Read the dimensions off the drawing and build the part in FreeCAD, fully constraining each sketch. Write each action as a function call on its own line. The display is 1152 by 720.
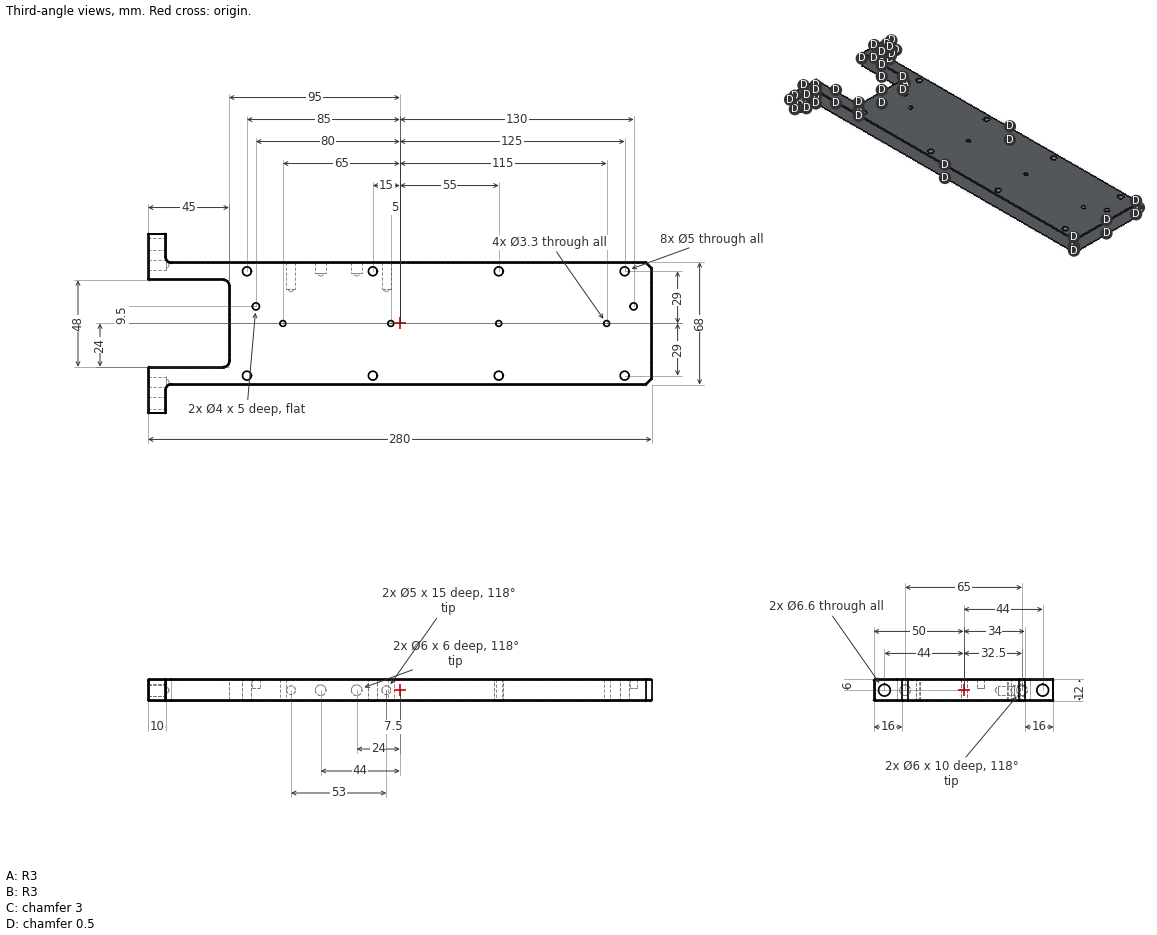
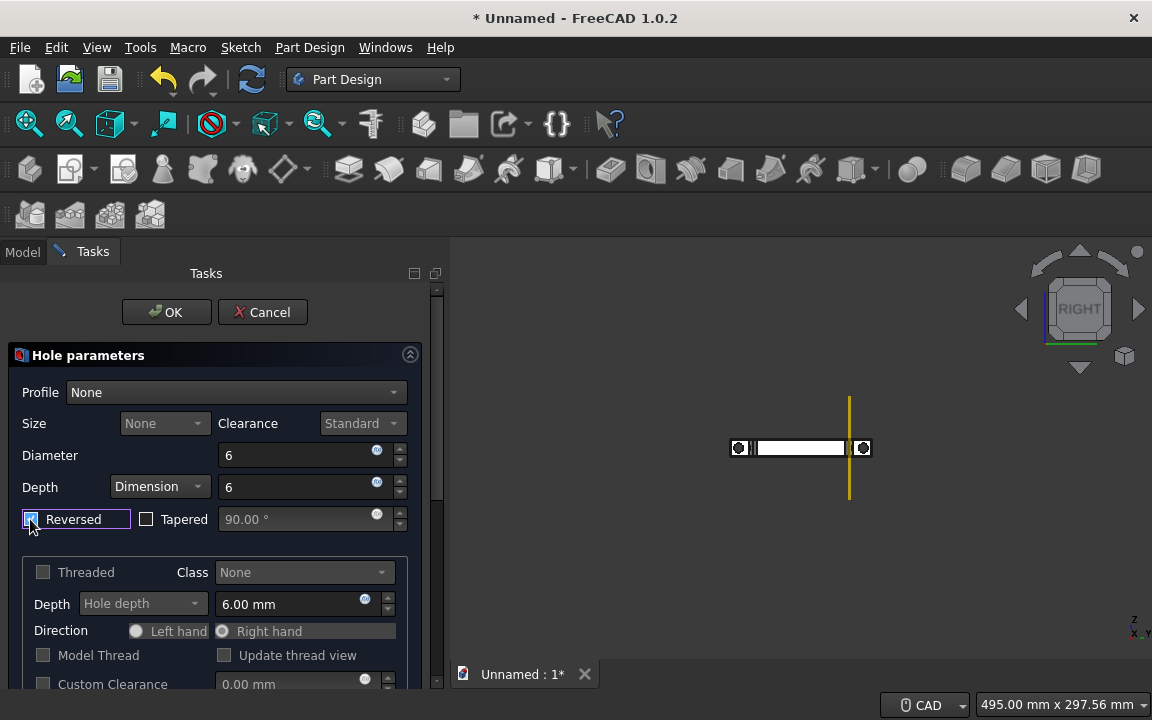
click(167, 312)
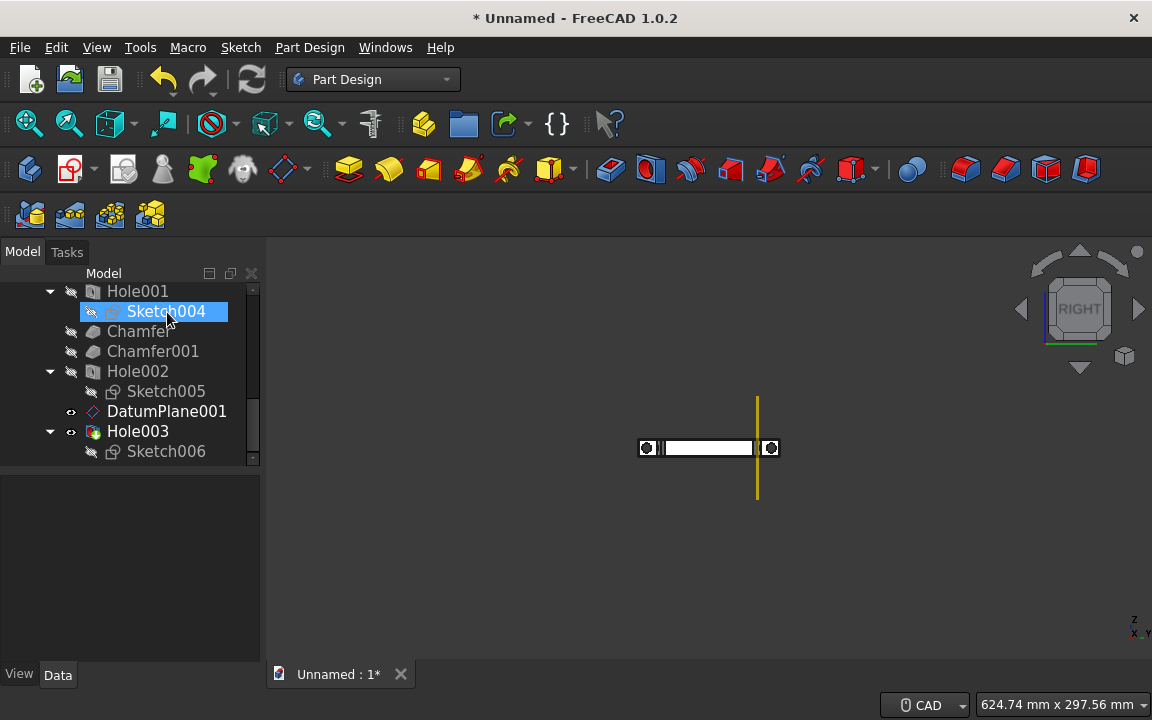
click(116, 412)
key(space)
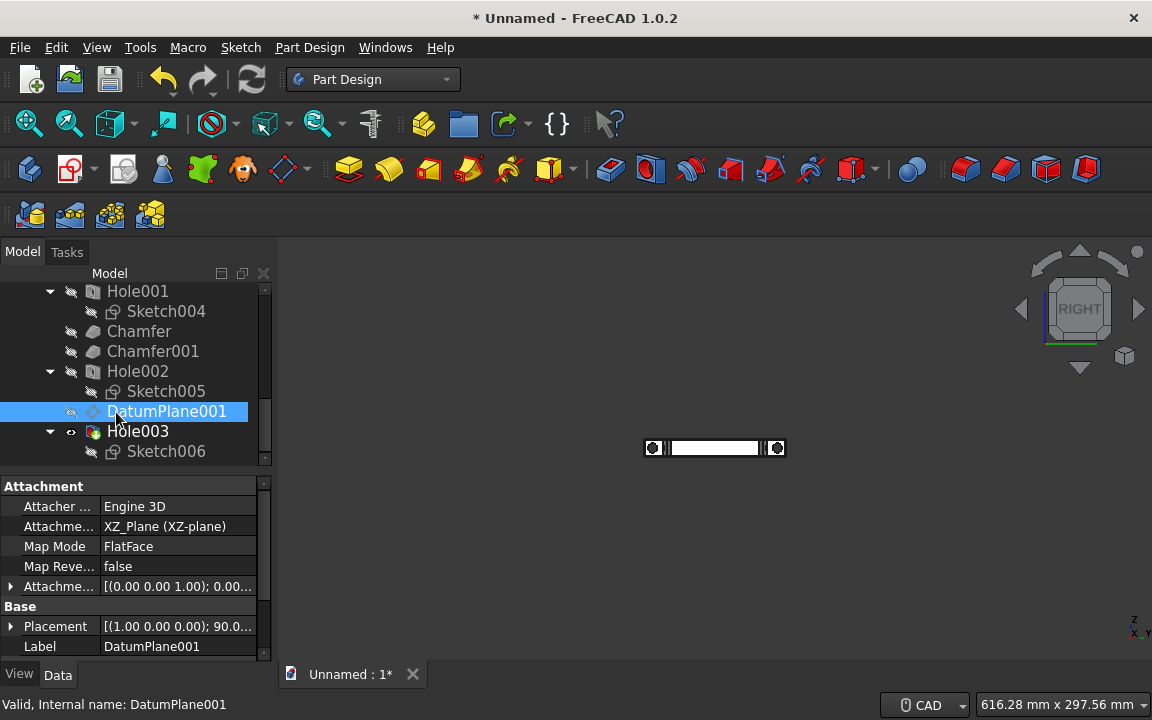
click(30, 124)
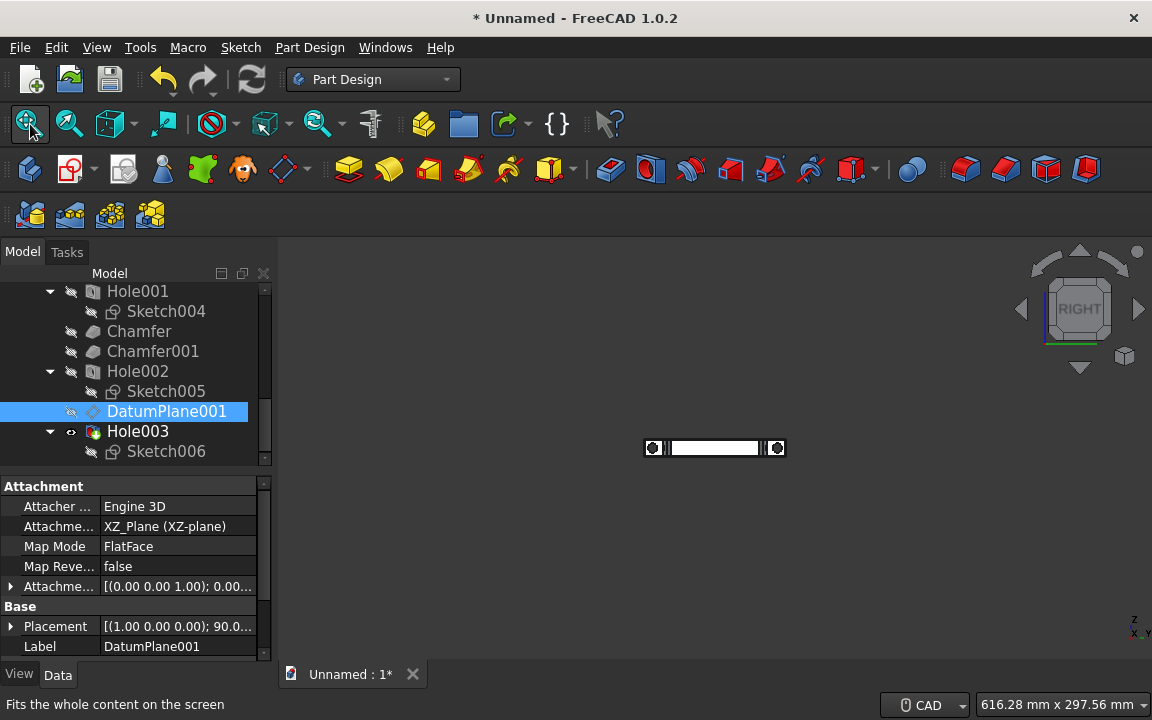
key(4)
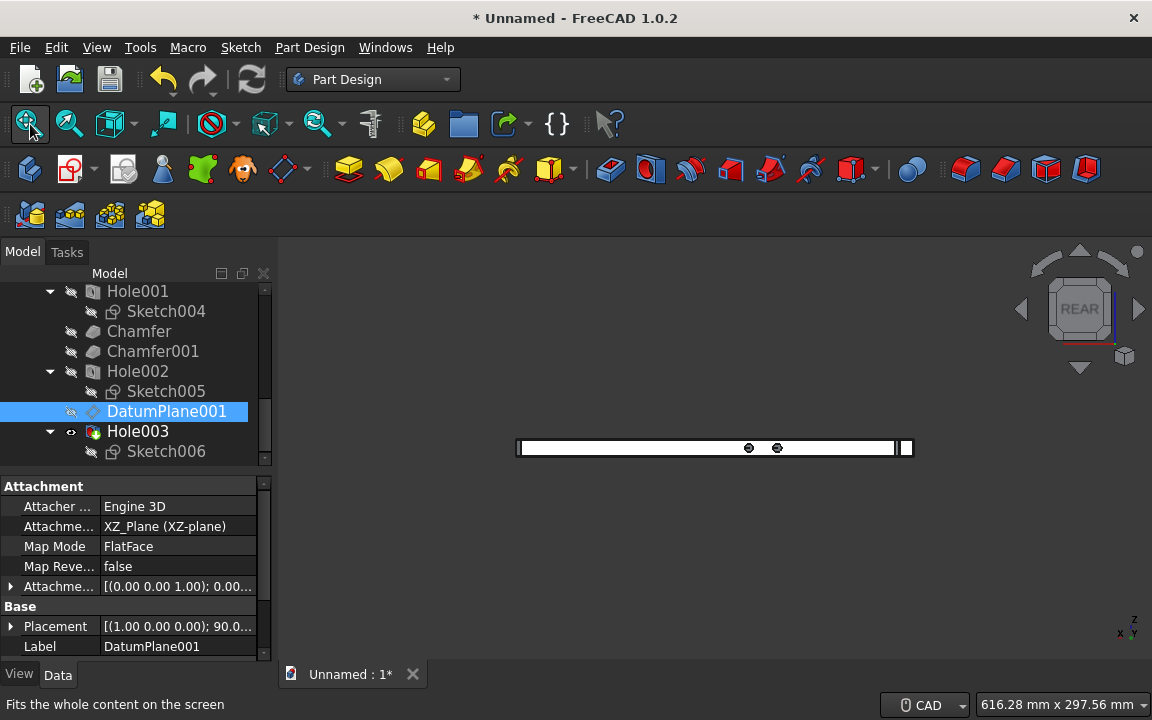
key(2)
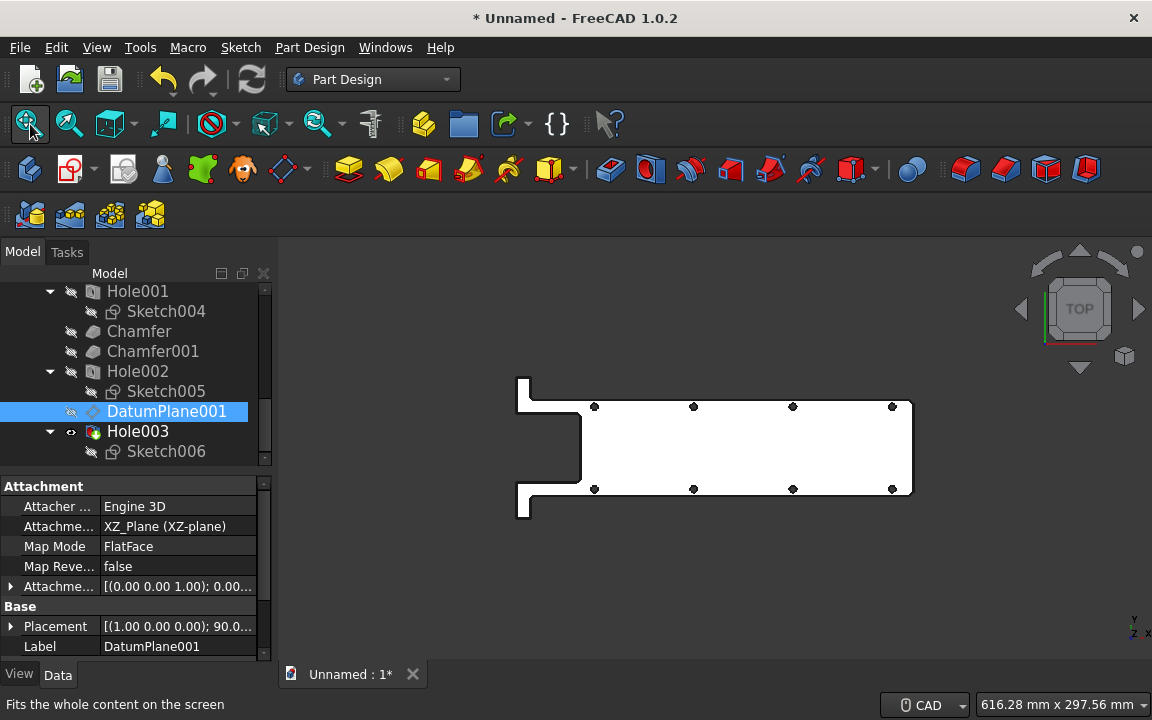
key(3)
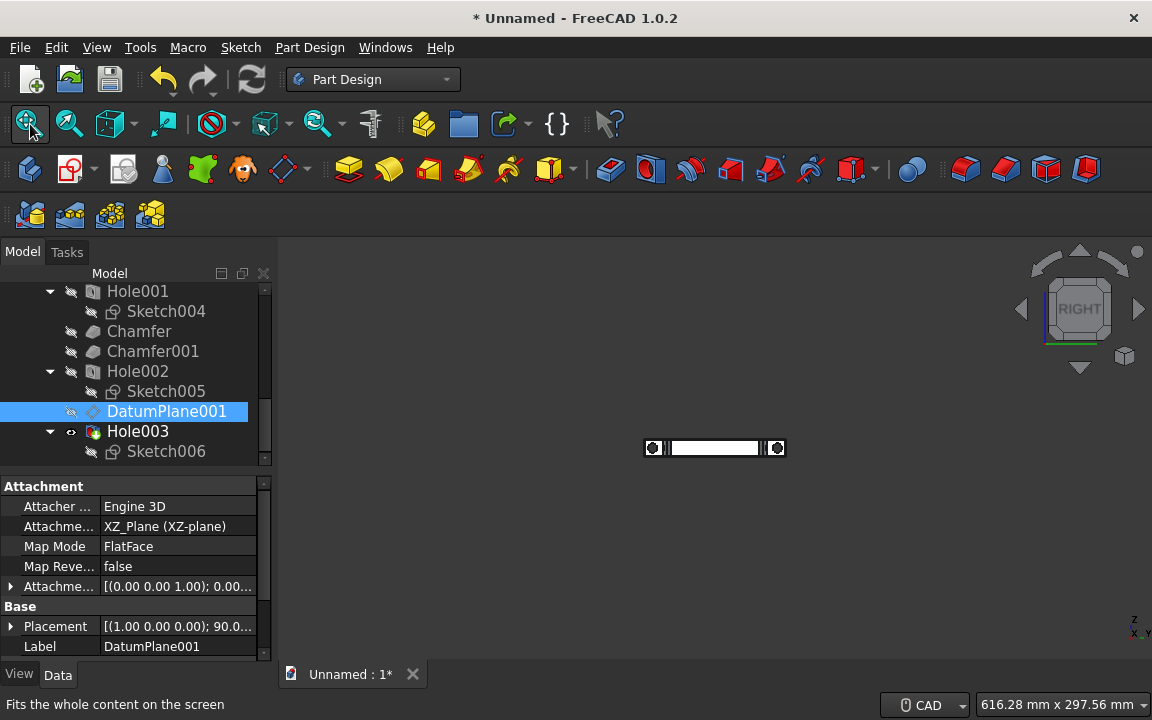
key(v)
key(f)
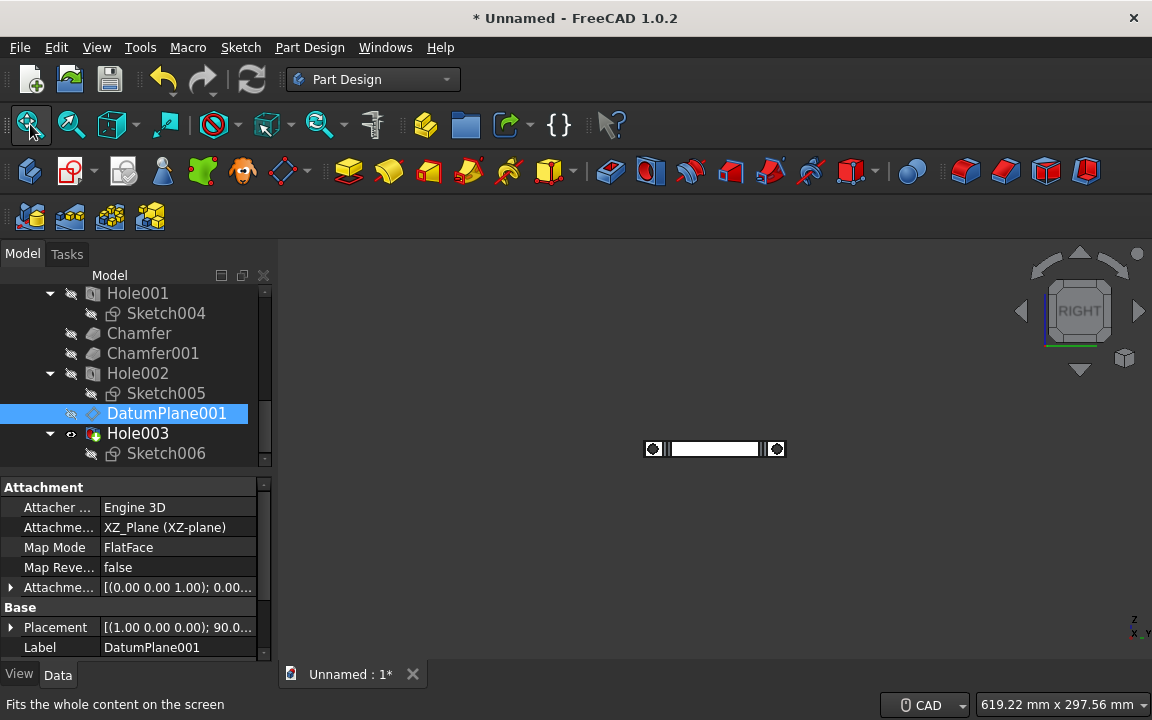
scroll(140, 369, down, 3)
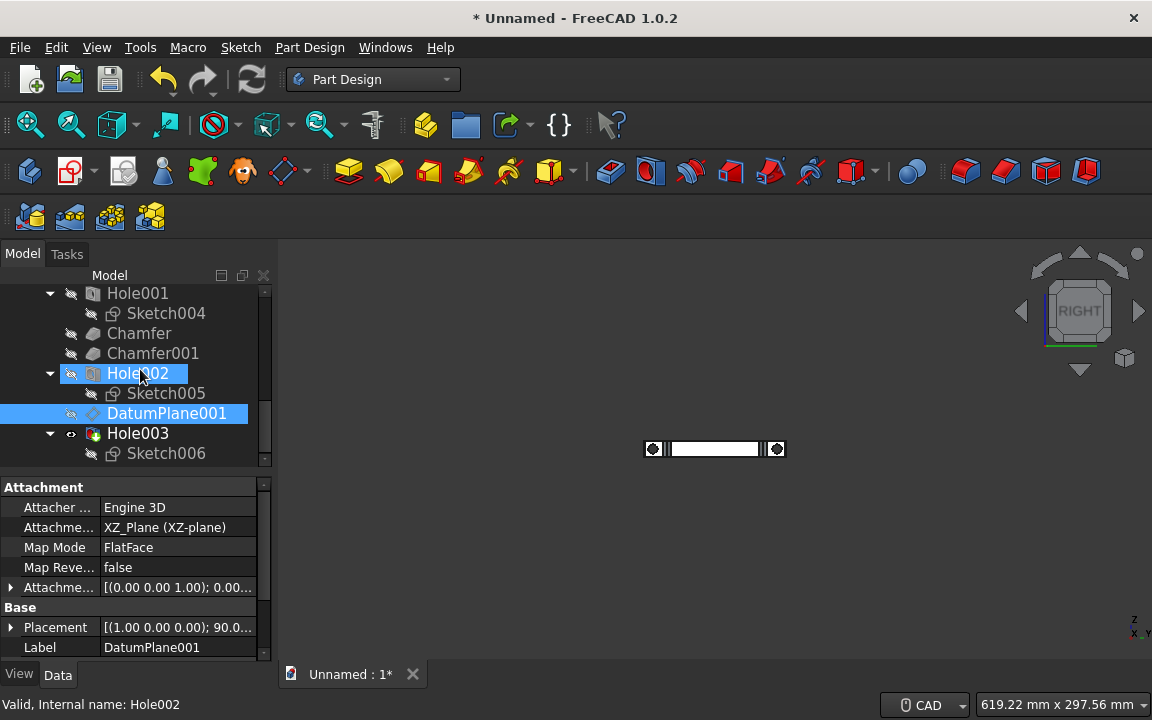
scroll(140, 369, up, 15)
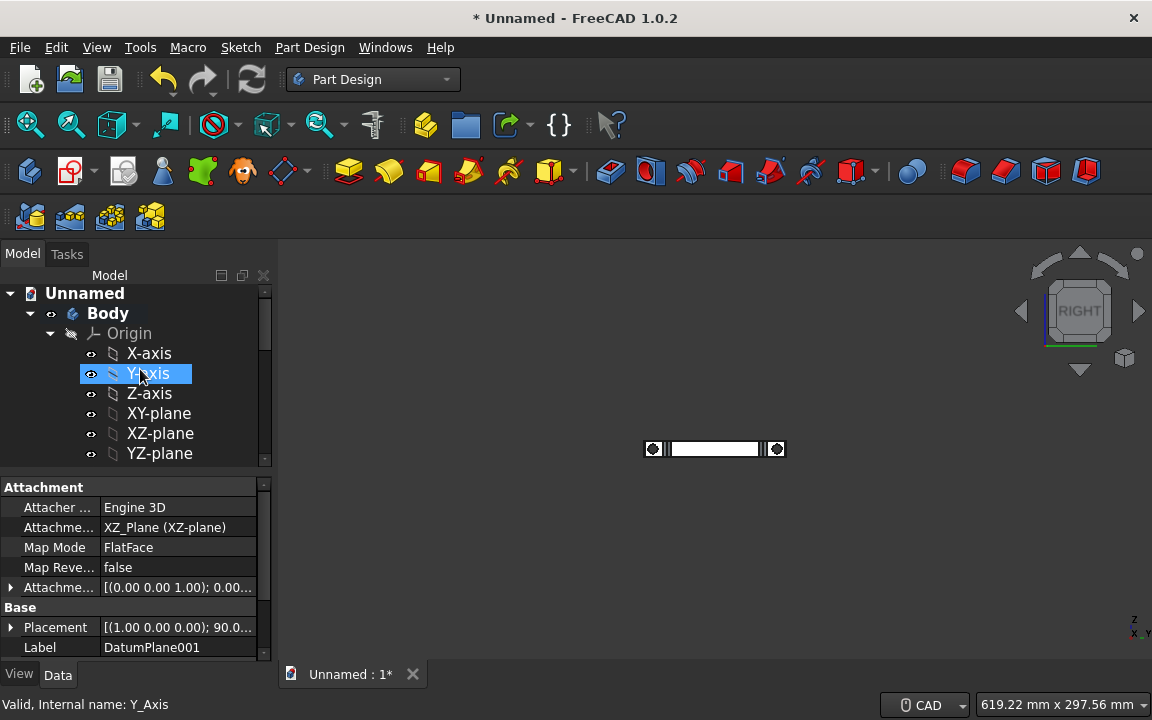
click(136, 434)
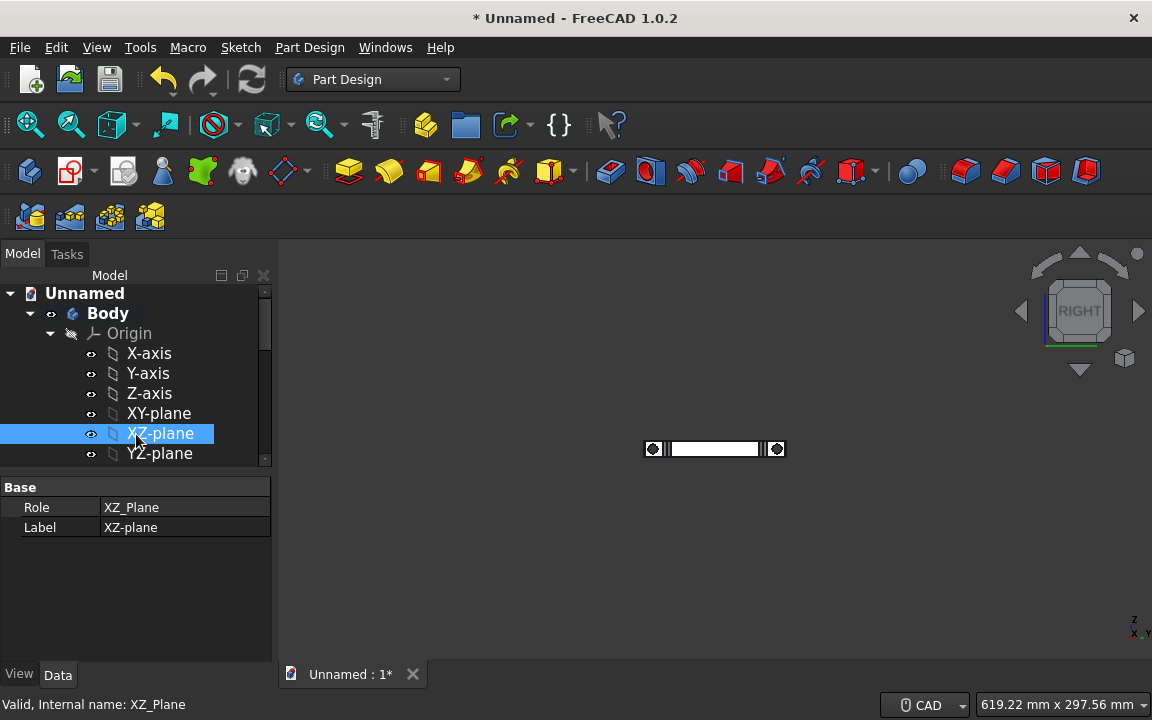
click(284, 172)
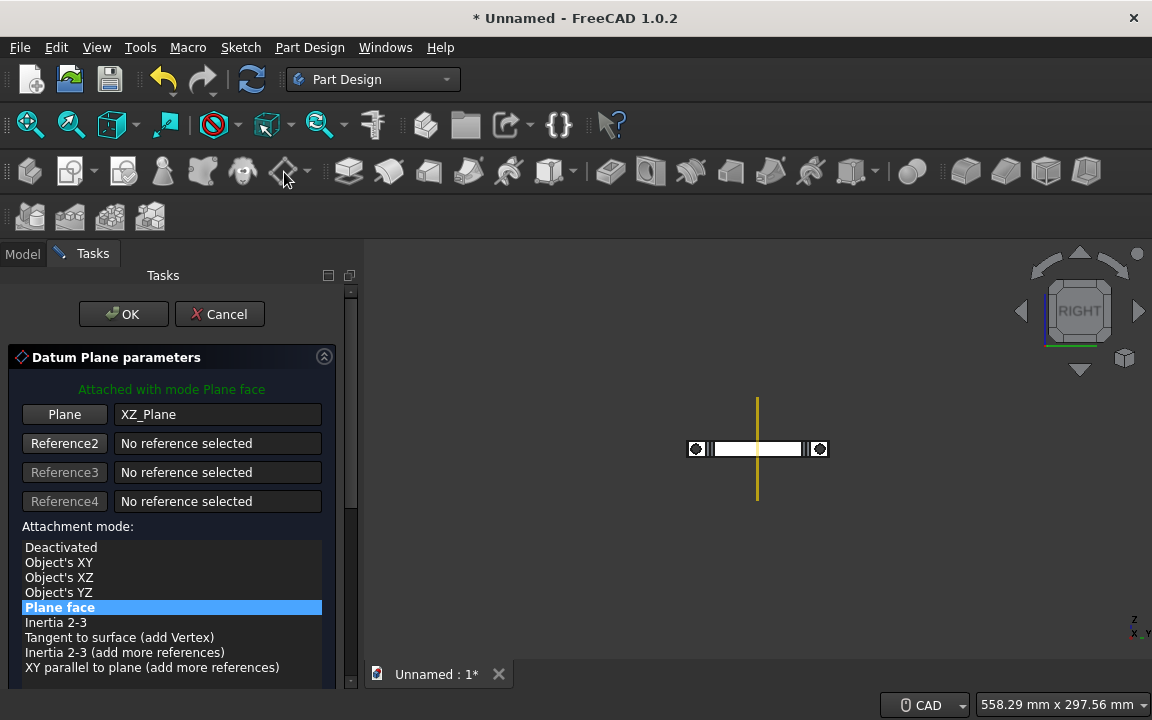
scroll(351, 486, down, 4)